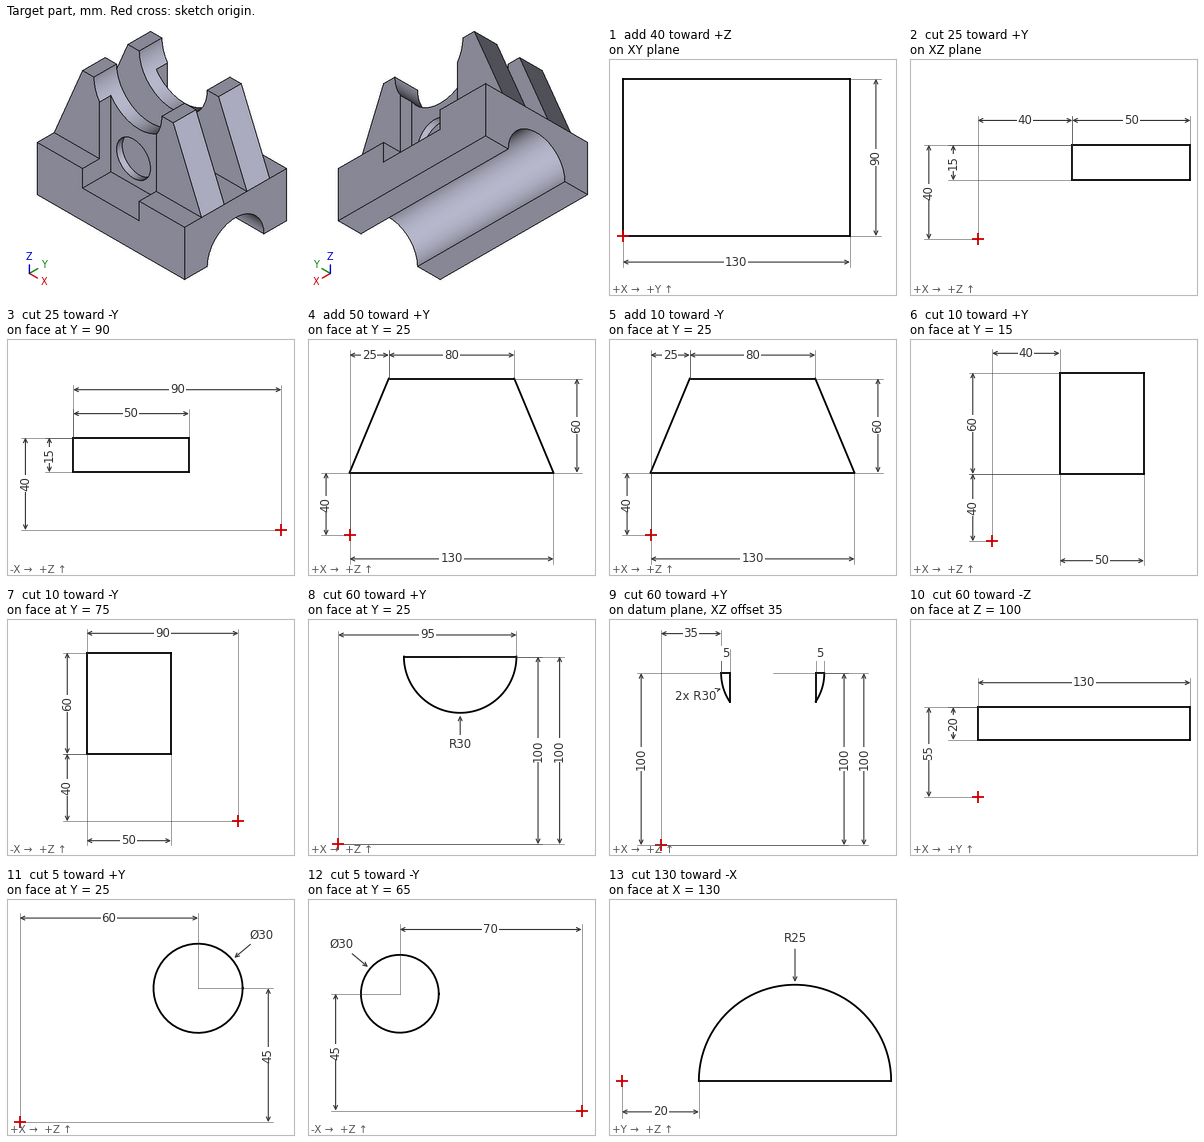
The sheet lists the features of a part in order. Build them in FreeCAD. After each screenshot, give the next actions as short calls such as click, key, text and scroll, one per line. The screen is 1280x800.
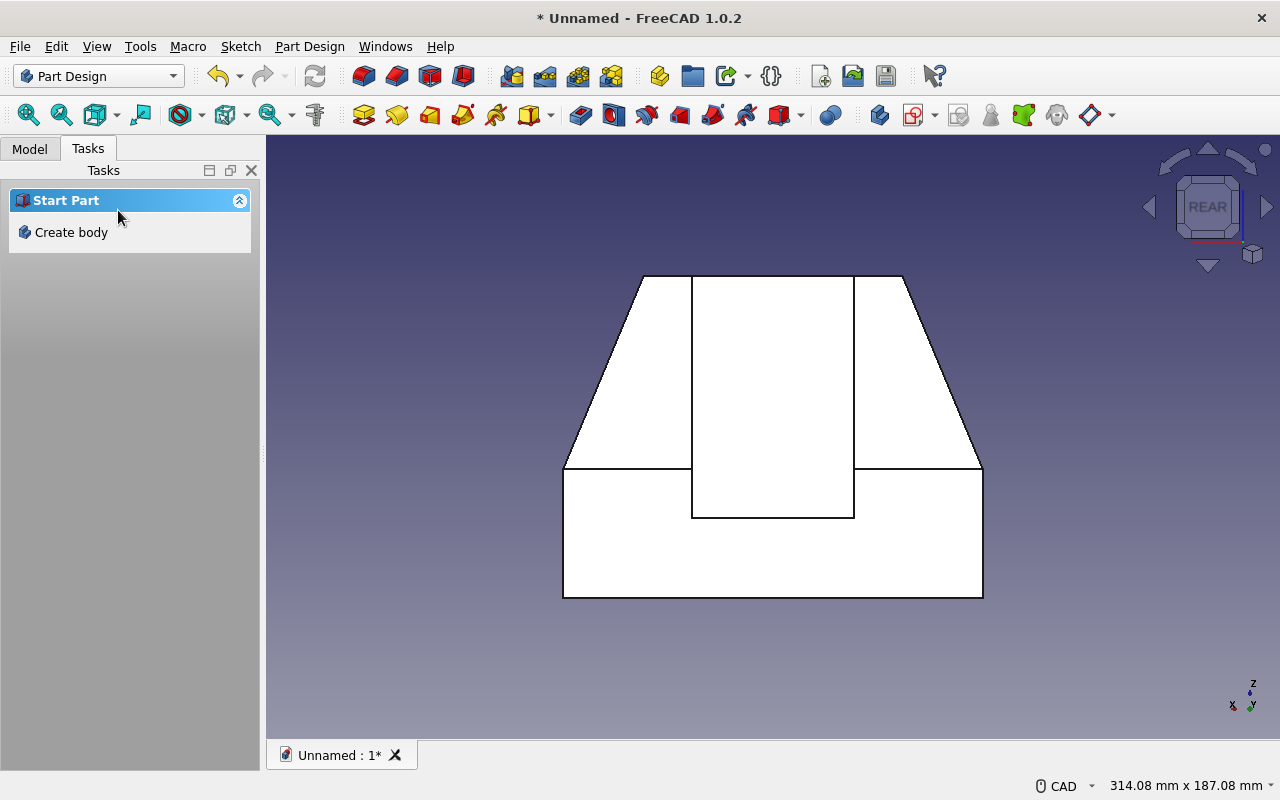
key(0)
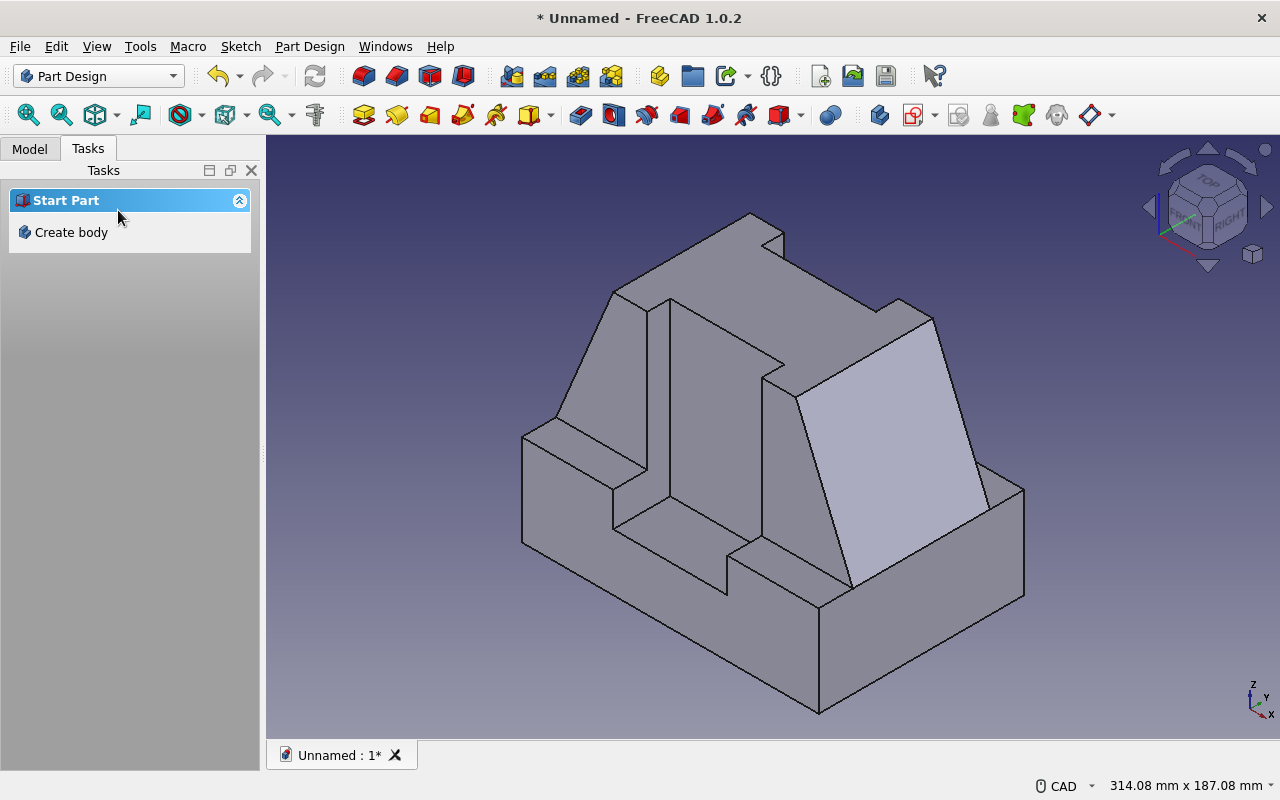
click(727, 401)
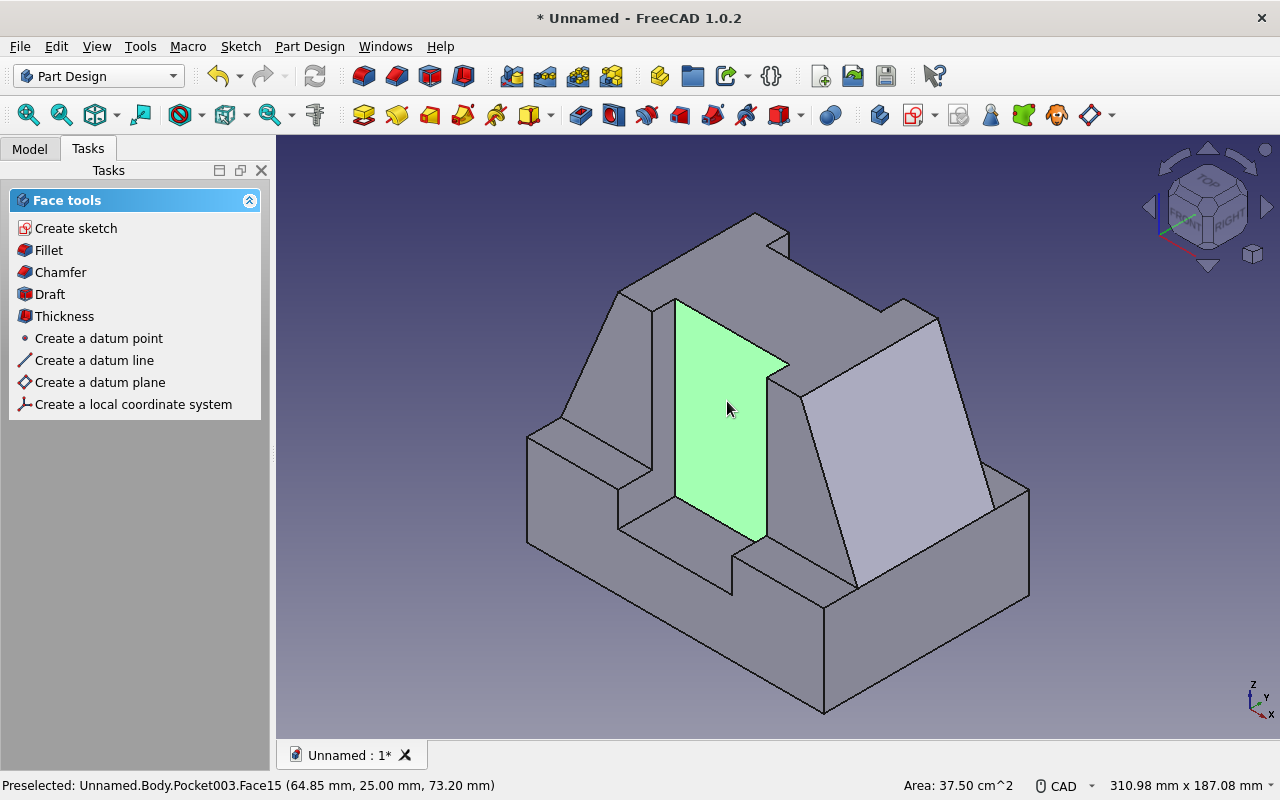
click(912, 116)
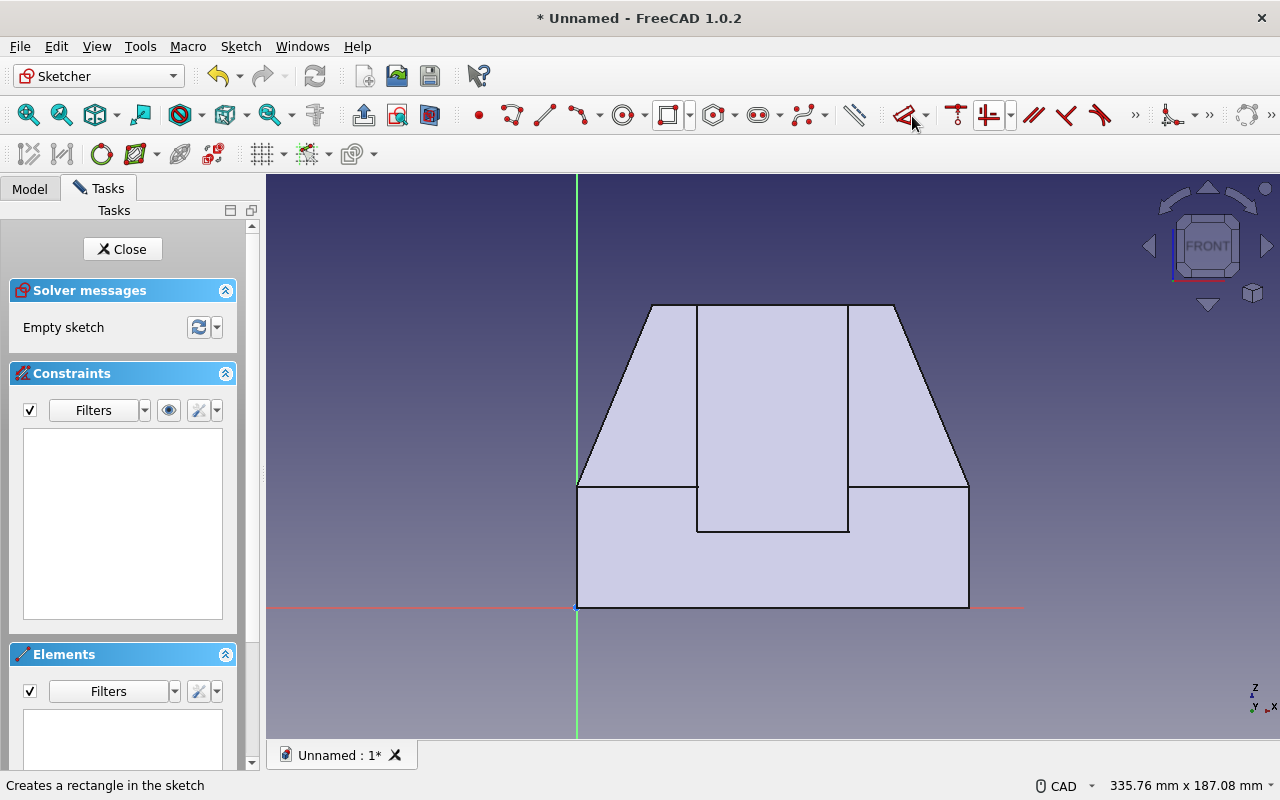
click(430, 116)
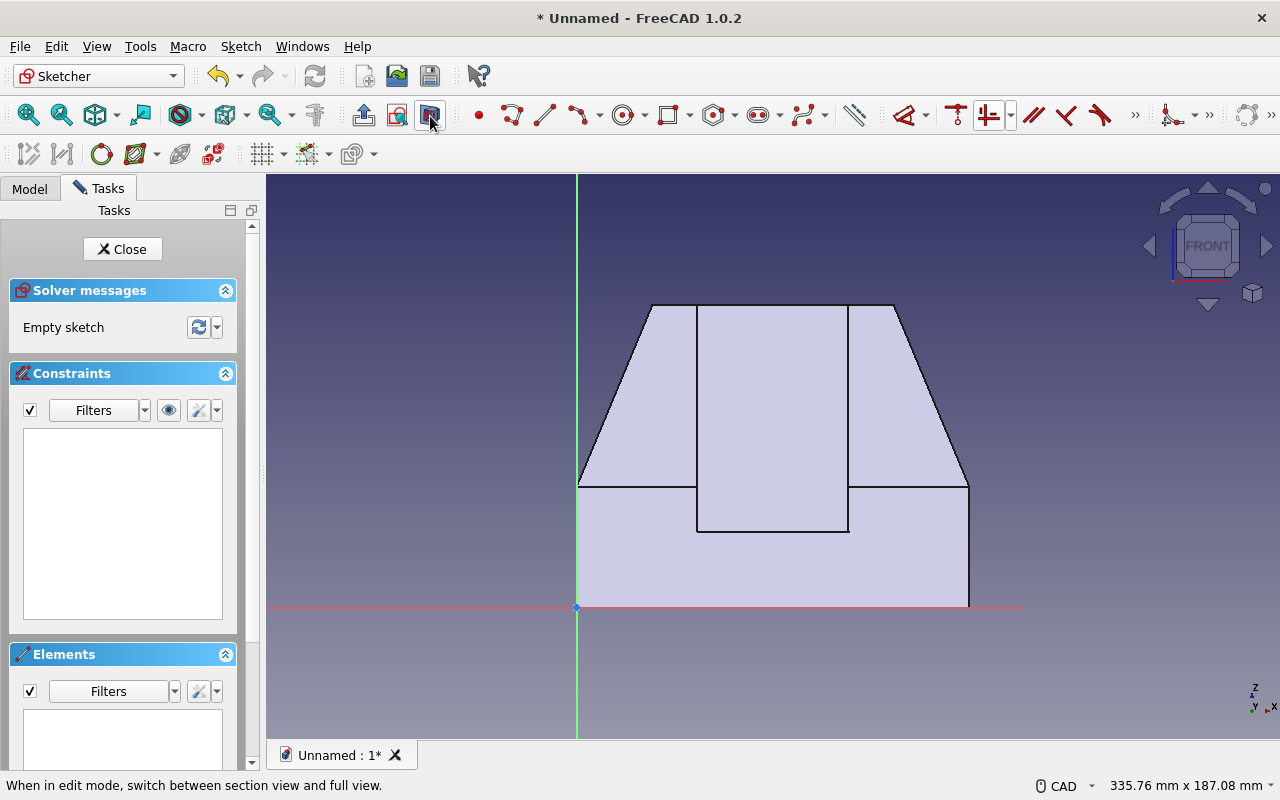
click(545, 116)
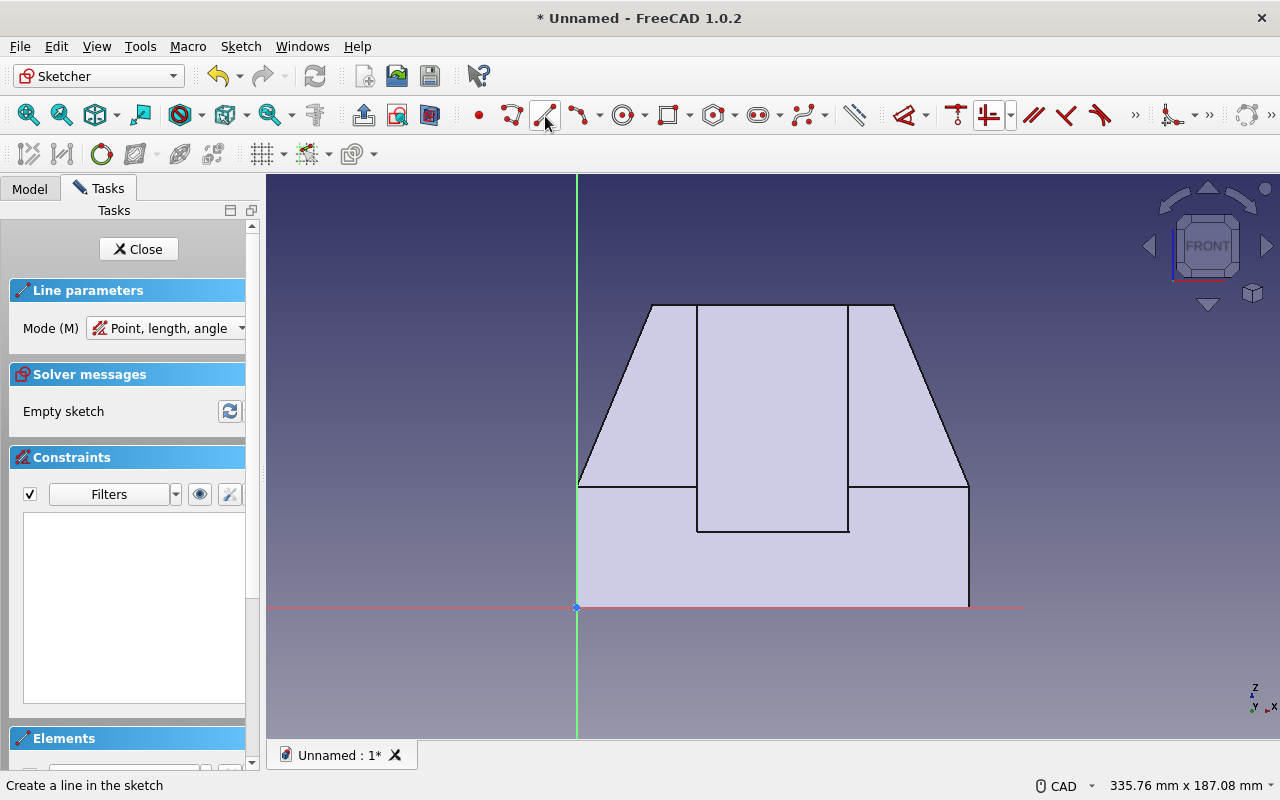
click(864, 305)
click(682, 305)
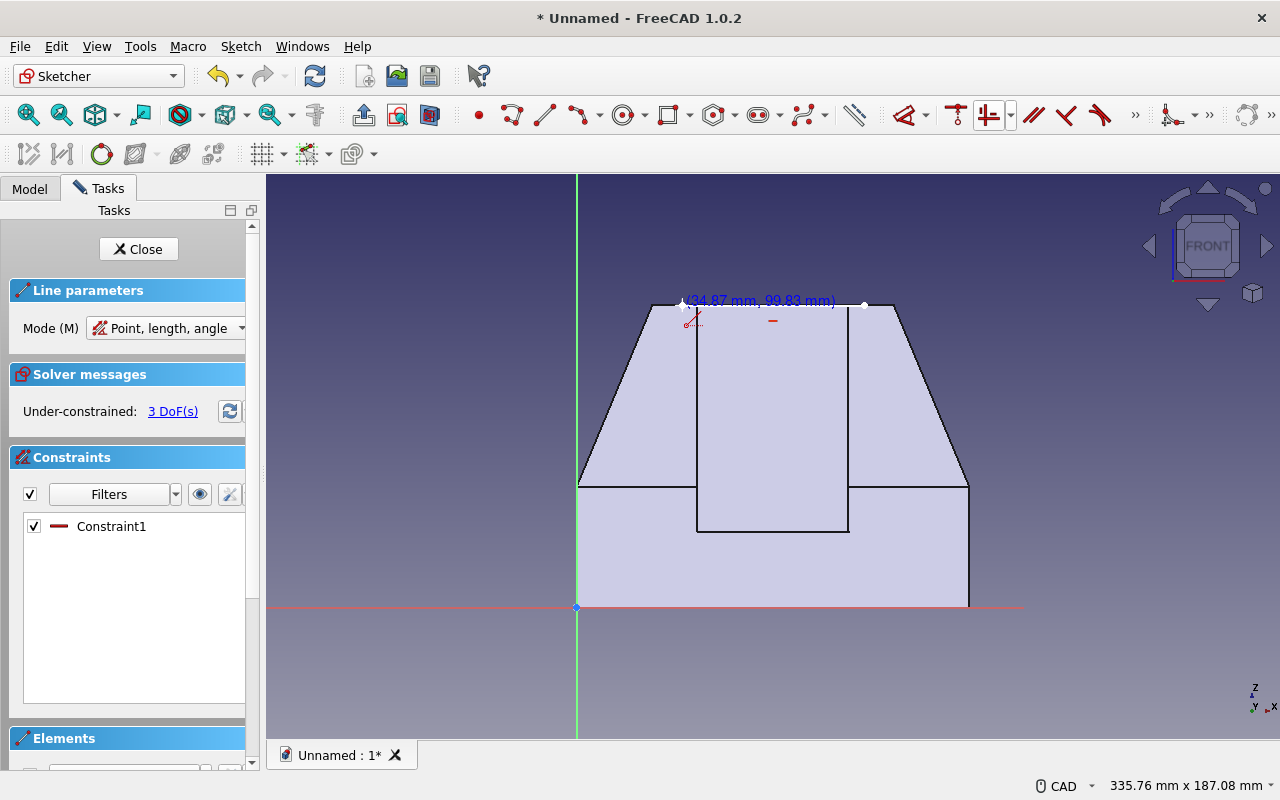
click(578, 116)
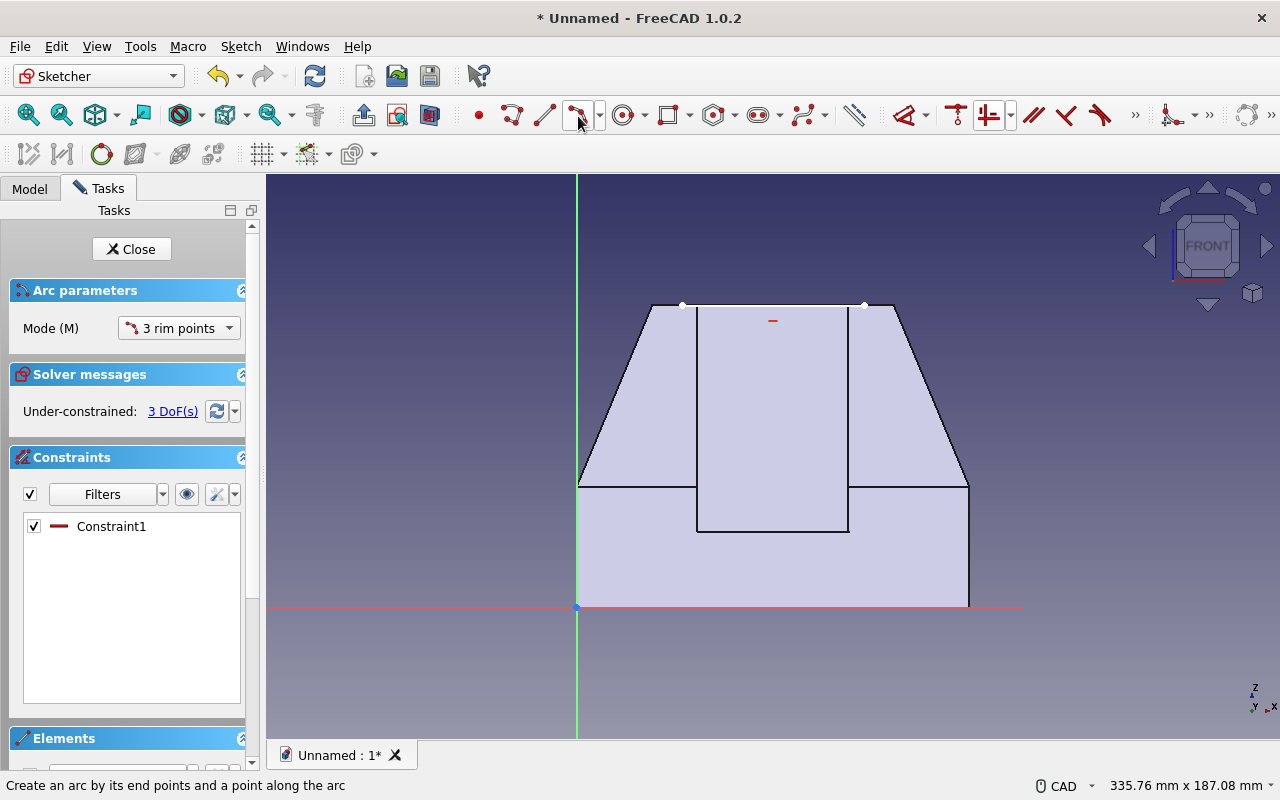
click(682, 306)
click(864, 306)
click(773, 396)
key(Escape)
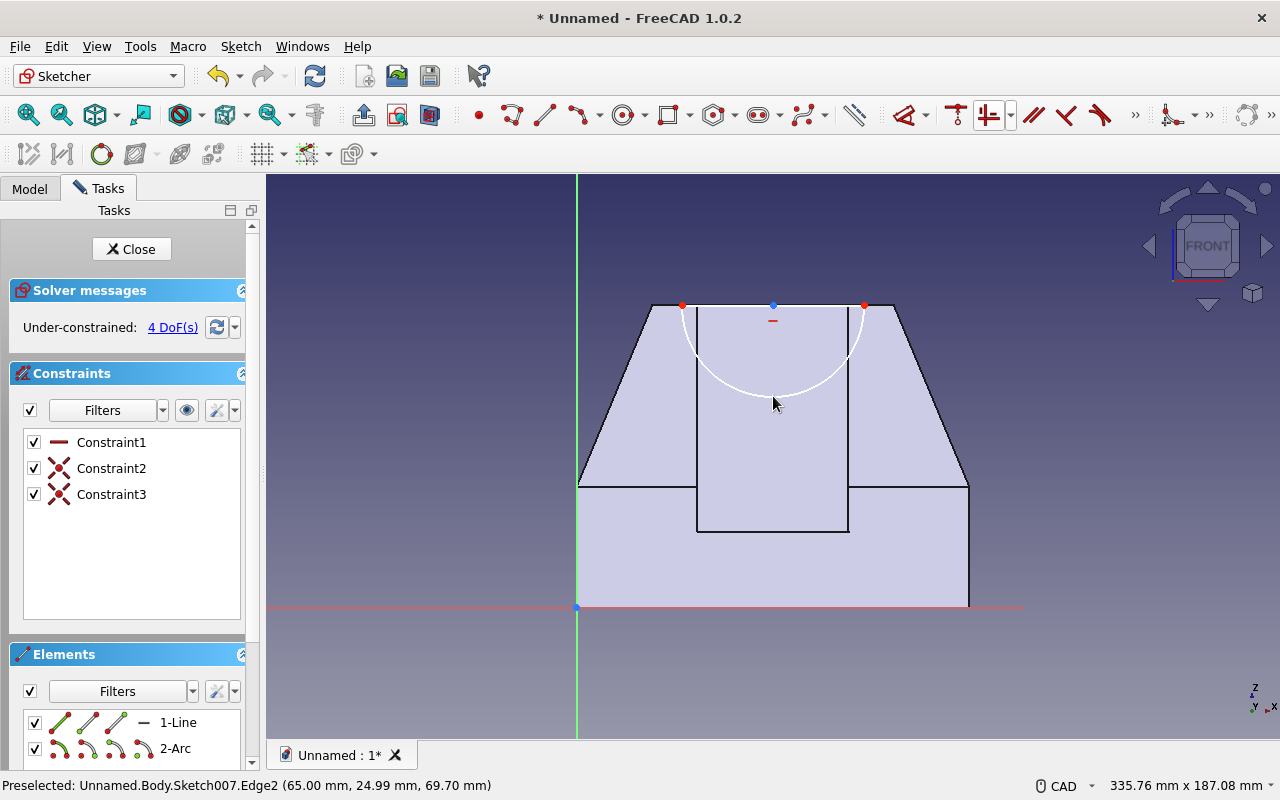
click(904, 116)